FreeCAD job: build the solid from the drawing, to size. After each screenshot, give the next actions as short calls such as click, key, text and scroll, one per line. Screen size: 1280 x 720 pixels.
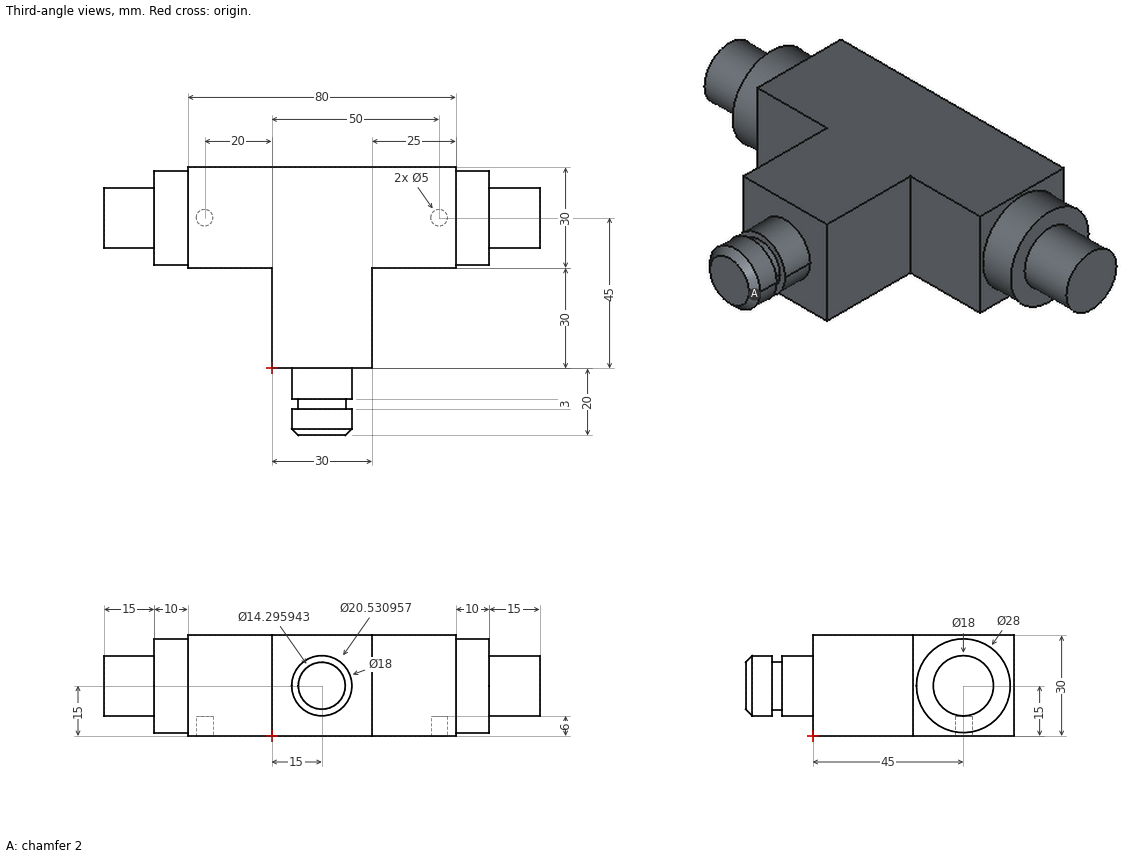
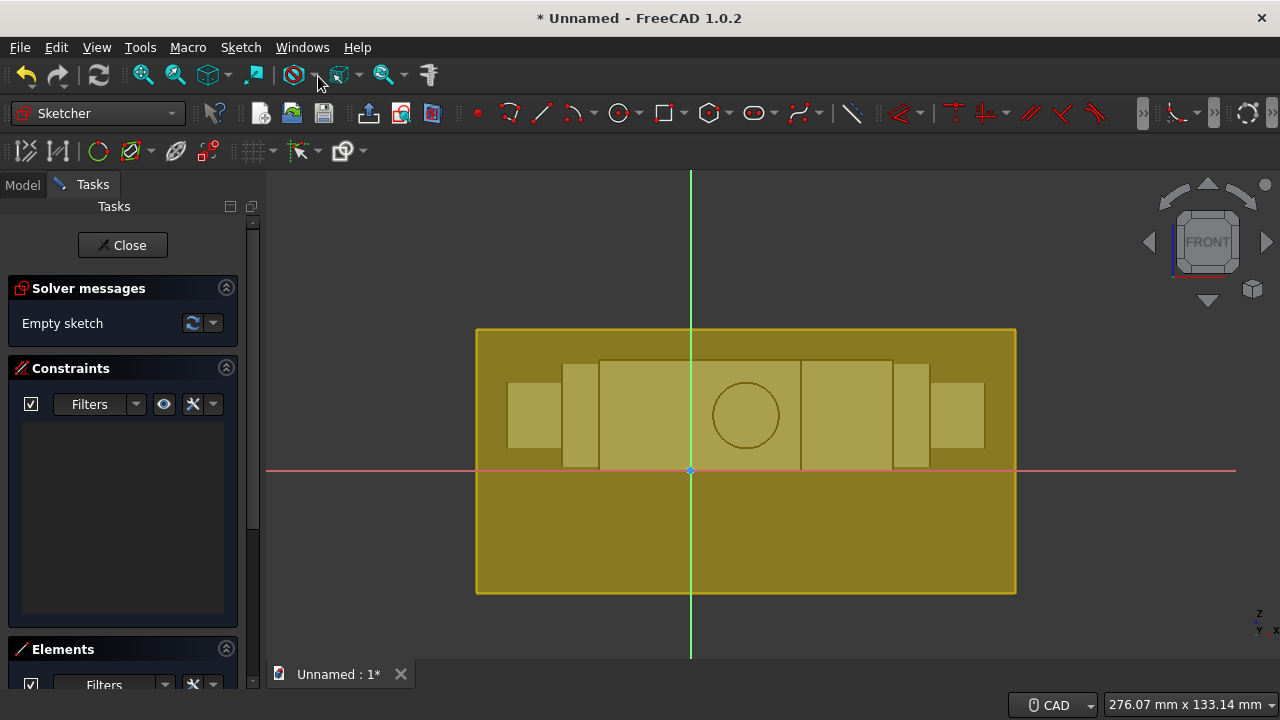
scroll(752, 428, up, 6)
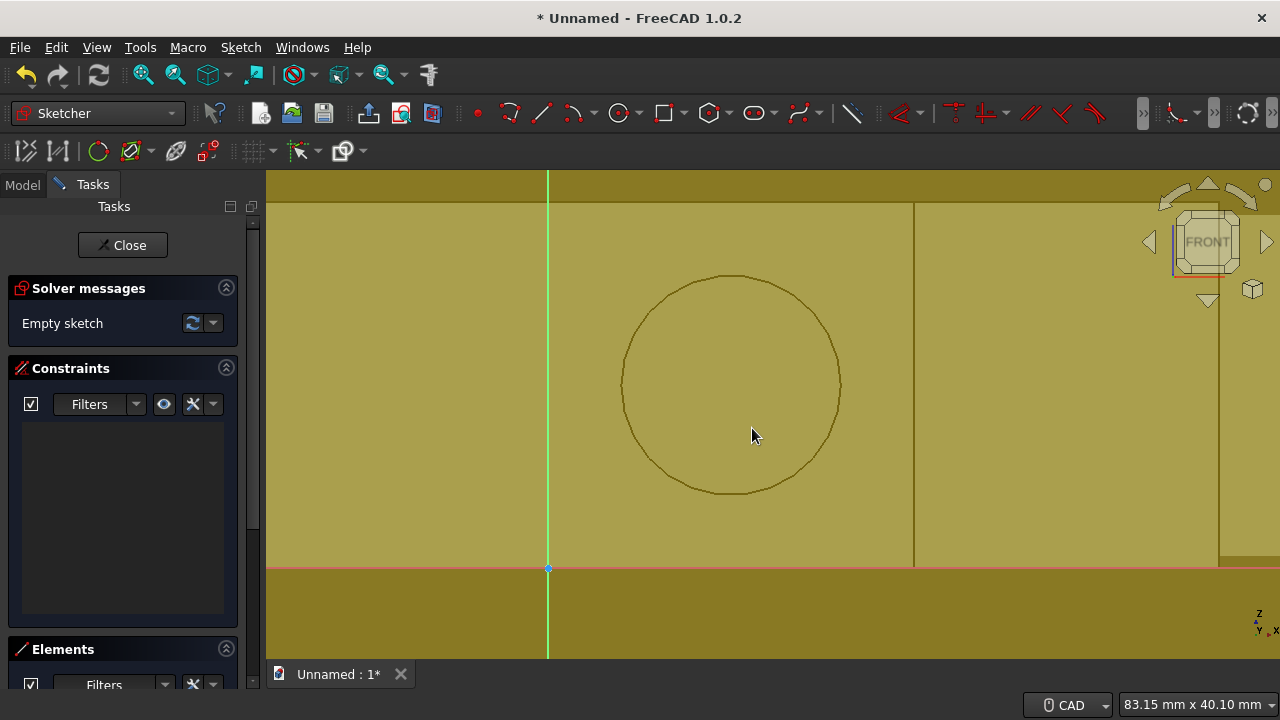
click(620, 114)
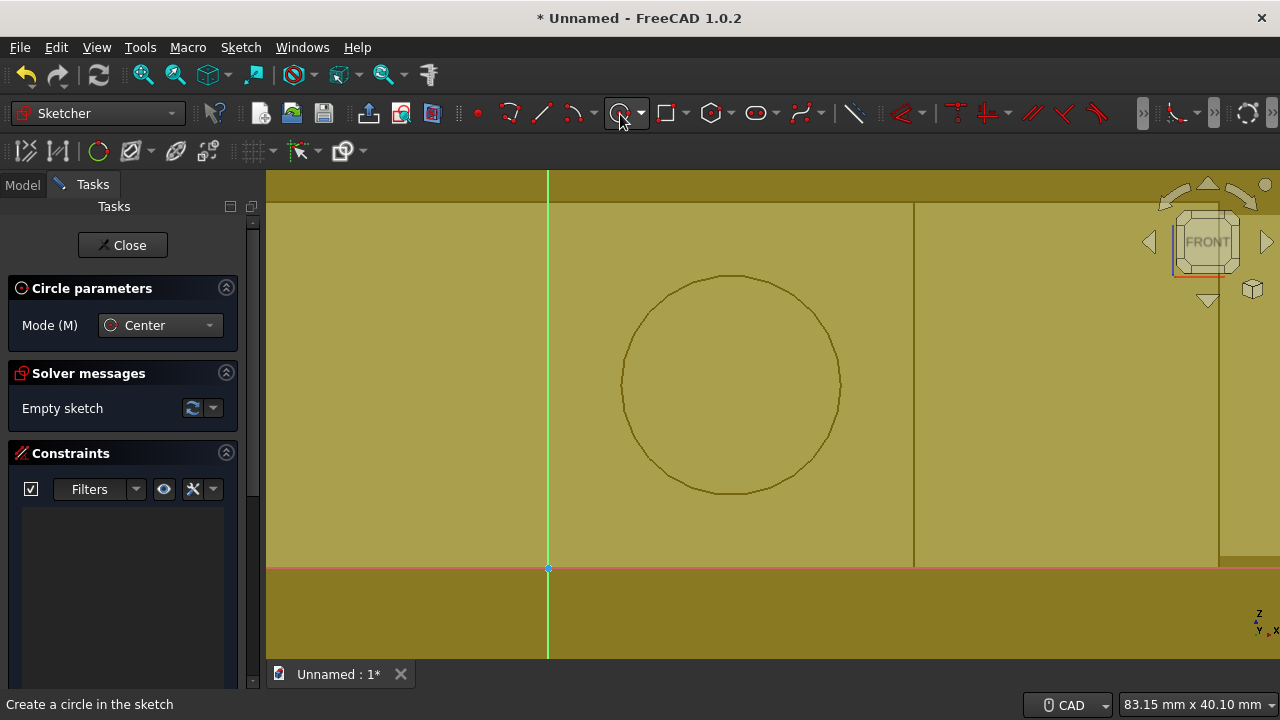
click(731, 385)
move(820, 297)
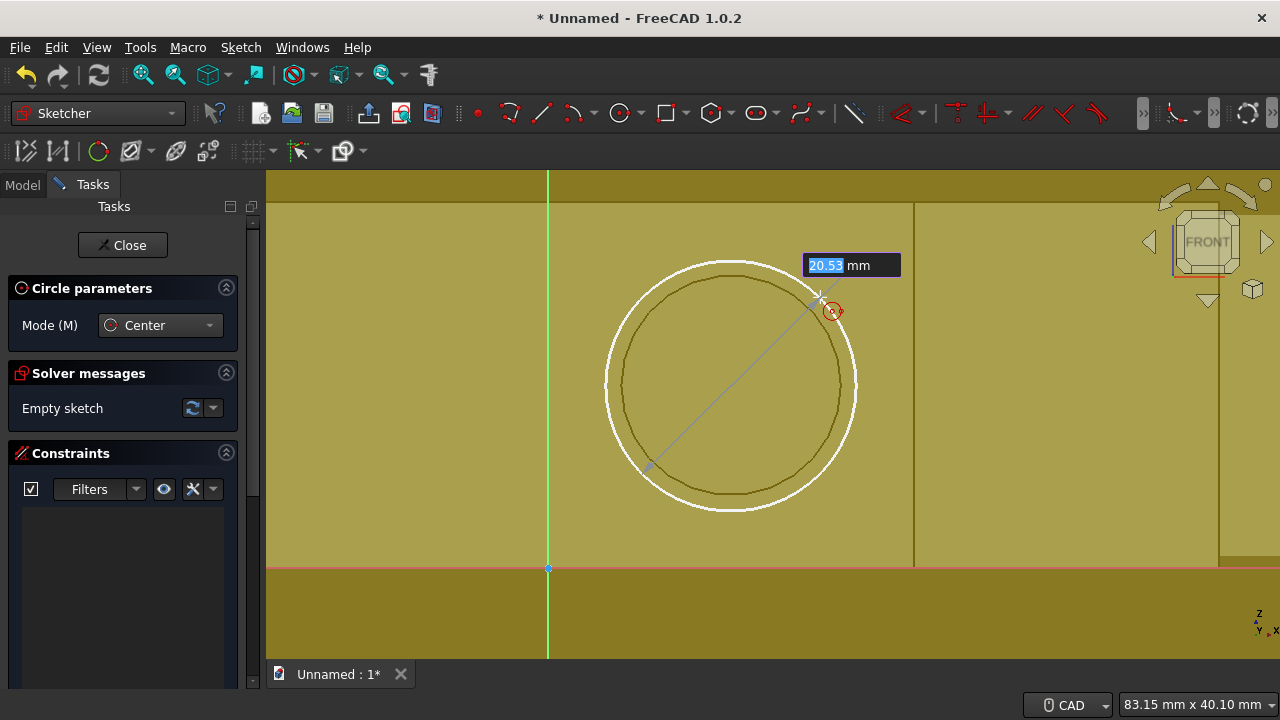
text(20.530957)
key(Return)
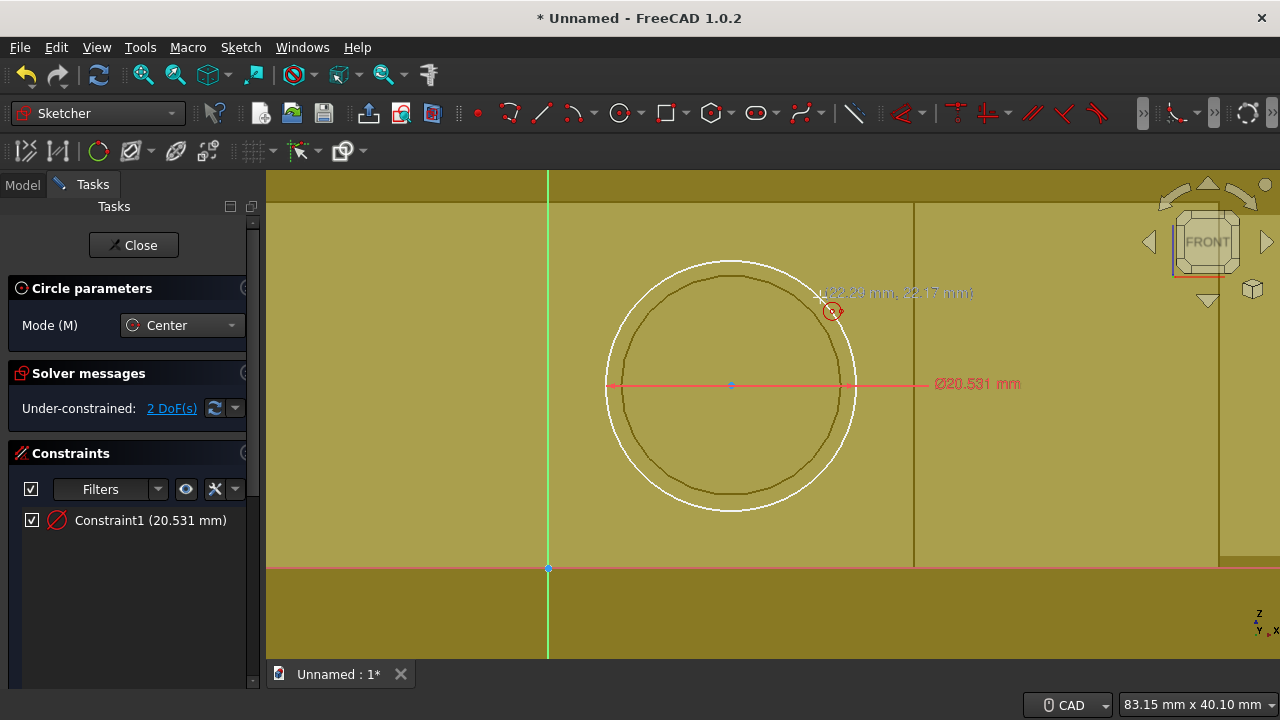
click(731, 386)
move(793, 324)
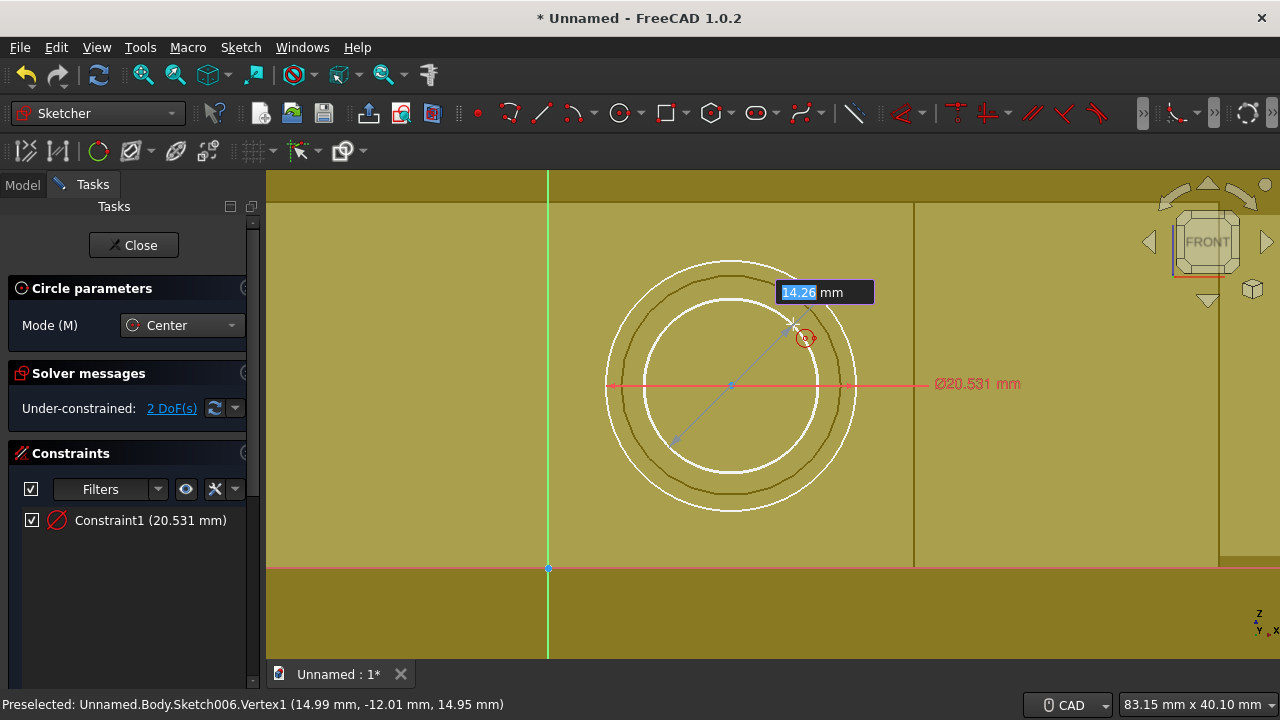
text(14.295943)
key(Return)
key(Escape)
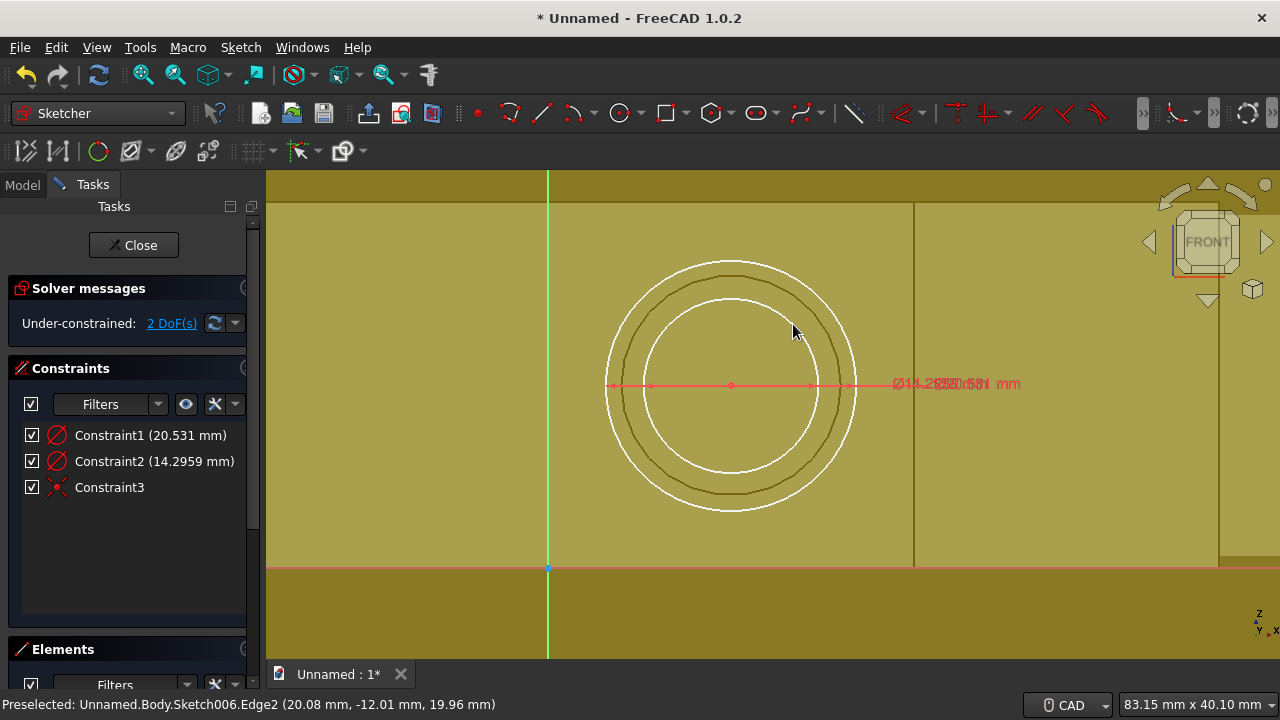
click(902, 114)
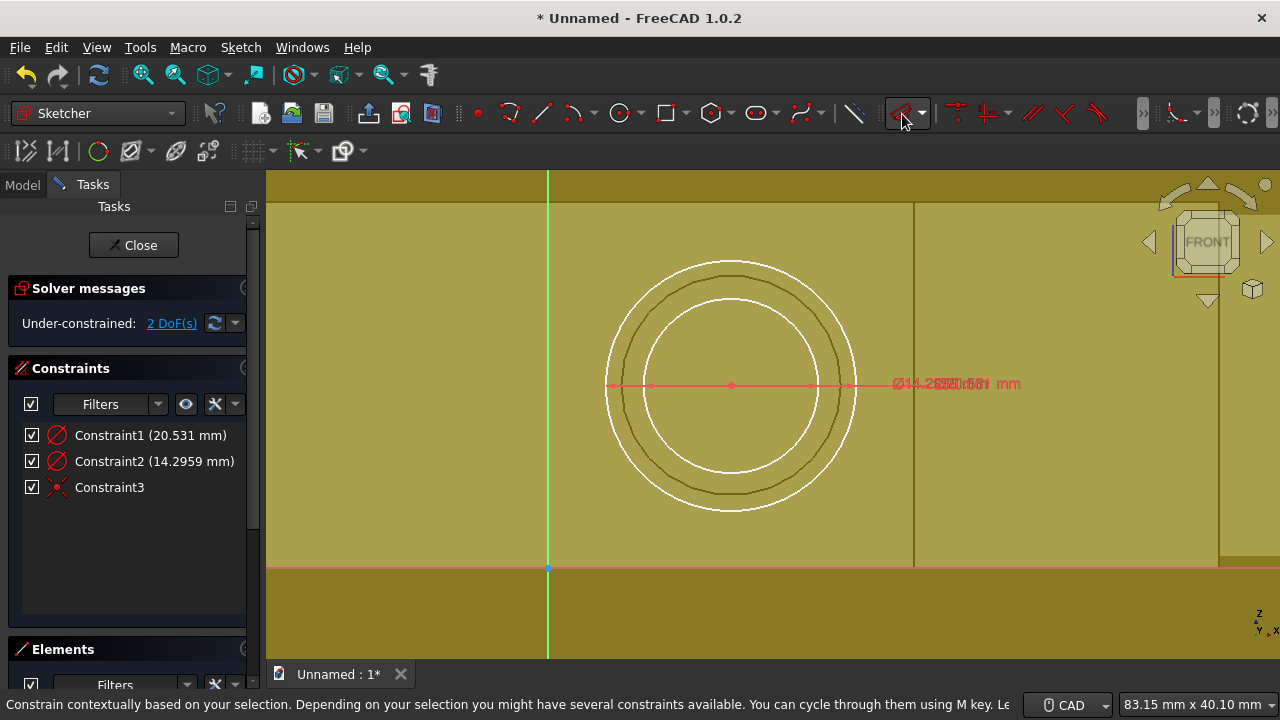
click(731, 386)
click(640, 602)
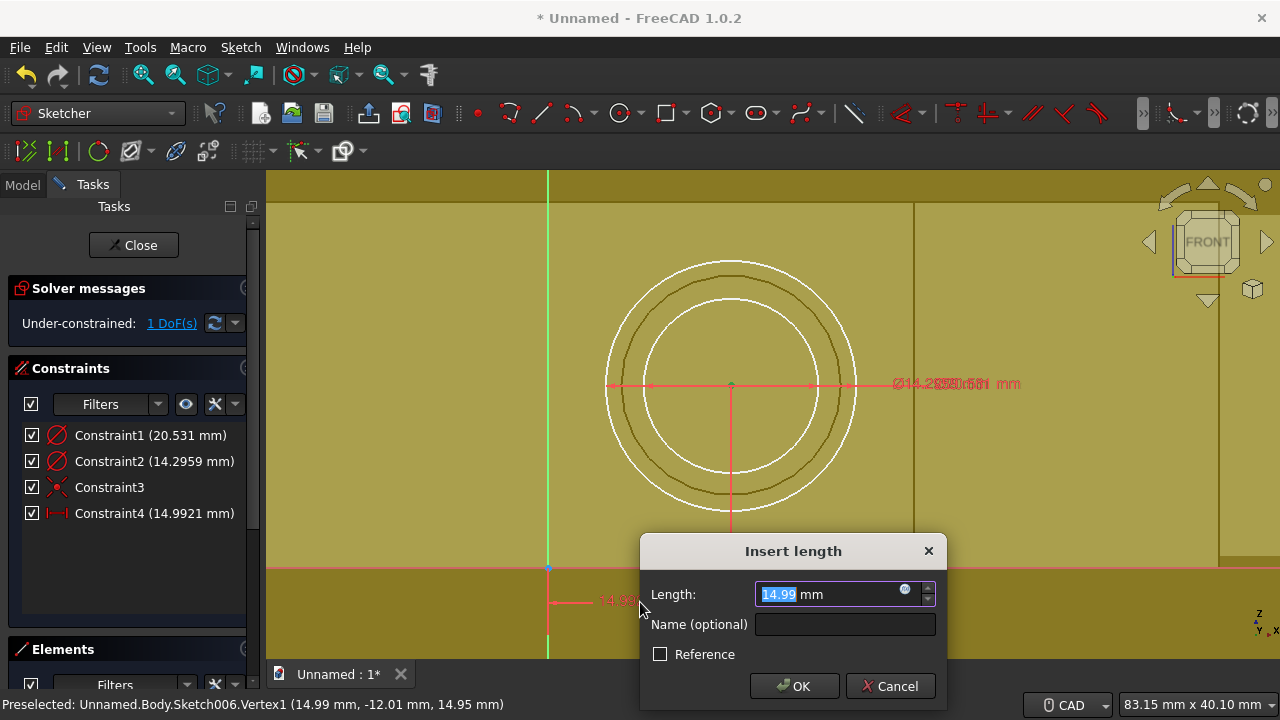
text(15)
key(Return)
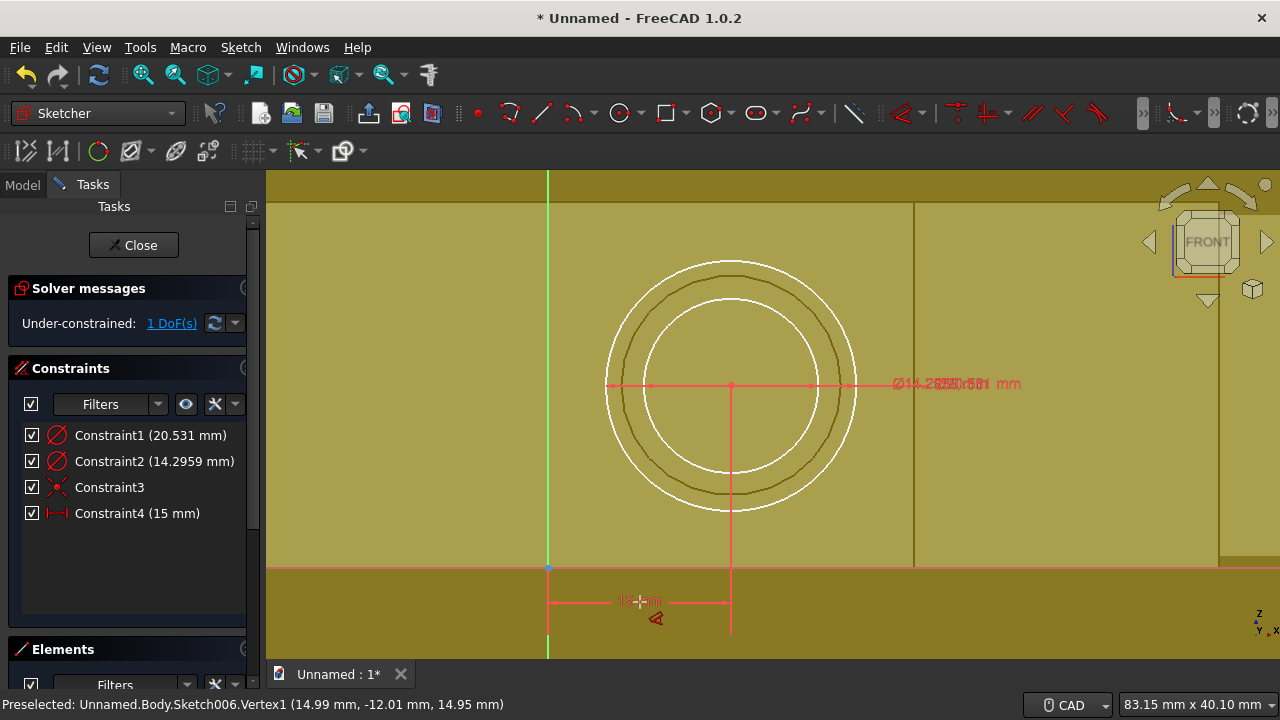
click(731, 386)
click(514, 477)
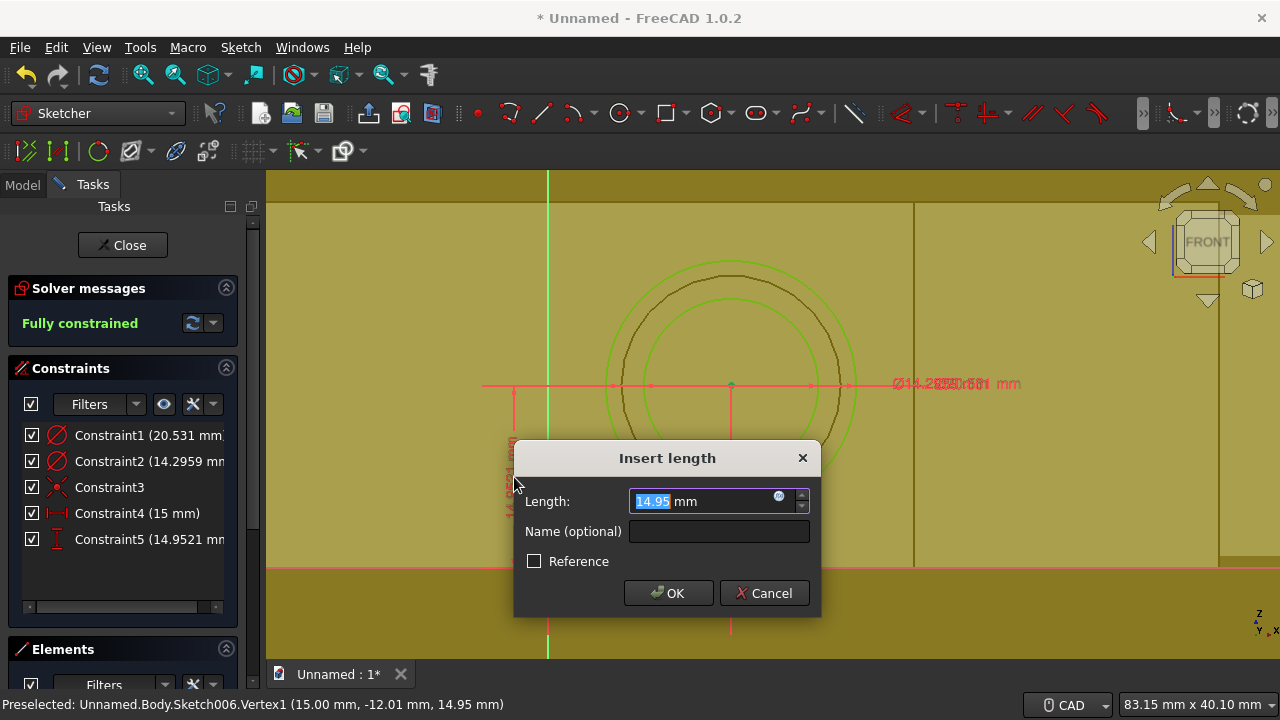
text(15)
key(Return)
key(Escape)